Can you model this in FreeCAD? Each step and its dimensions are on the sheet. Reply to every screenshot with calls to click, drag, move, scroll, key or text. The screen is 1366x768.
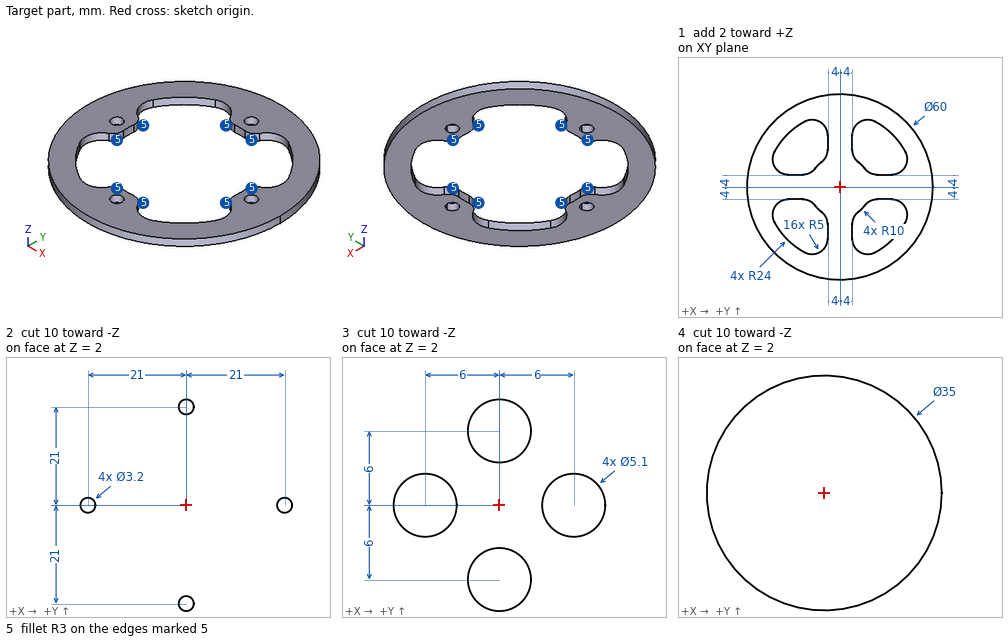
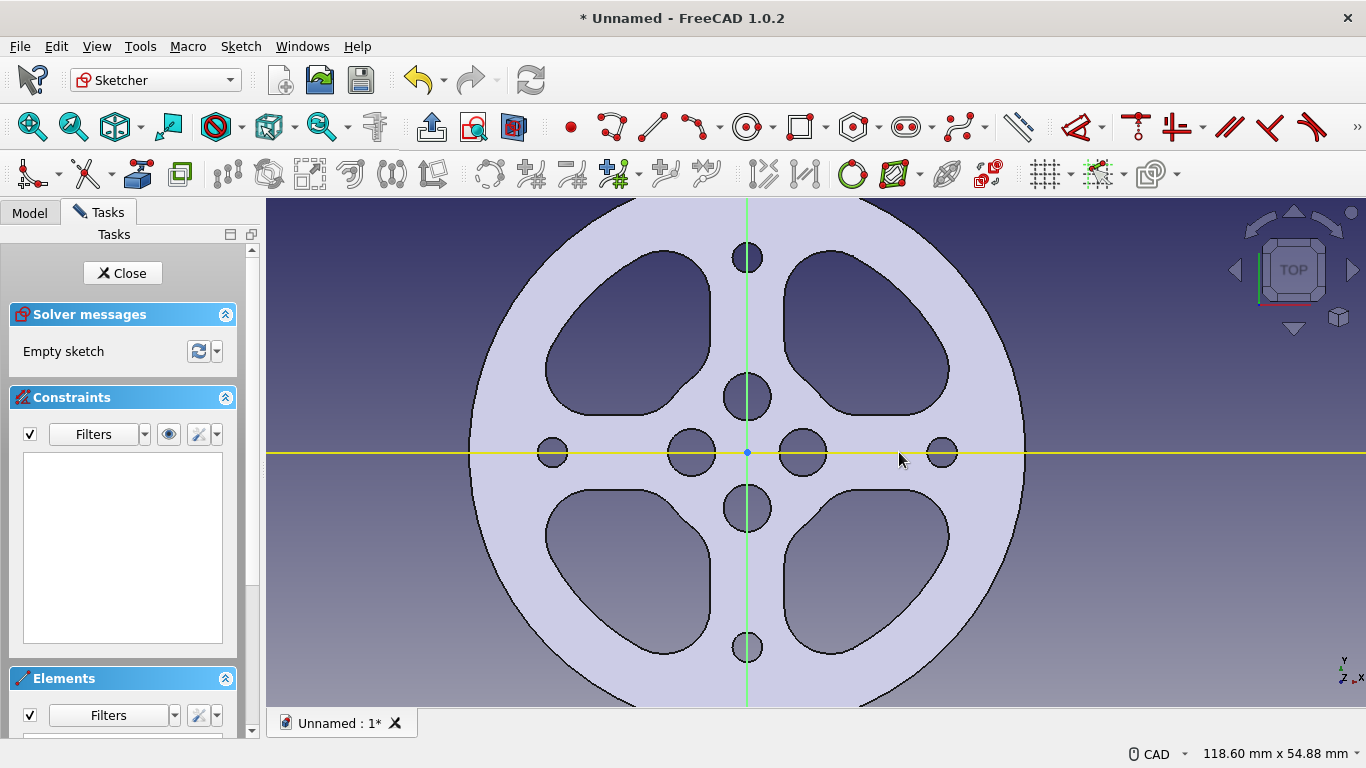
click(746, 128)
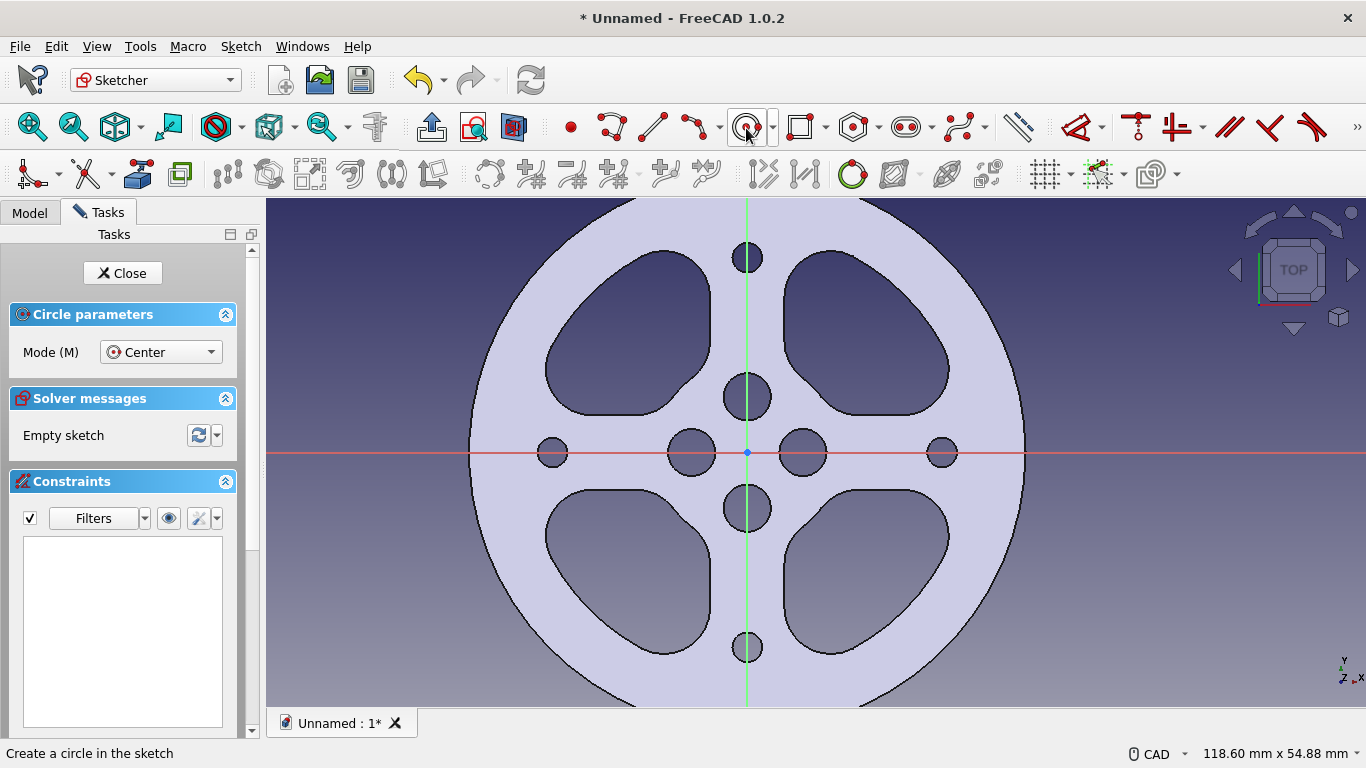
click(747, 452)
click(862, 338)
key(Escape)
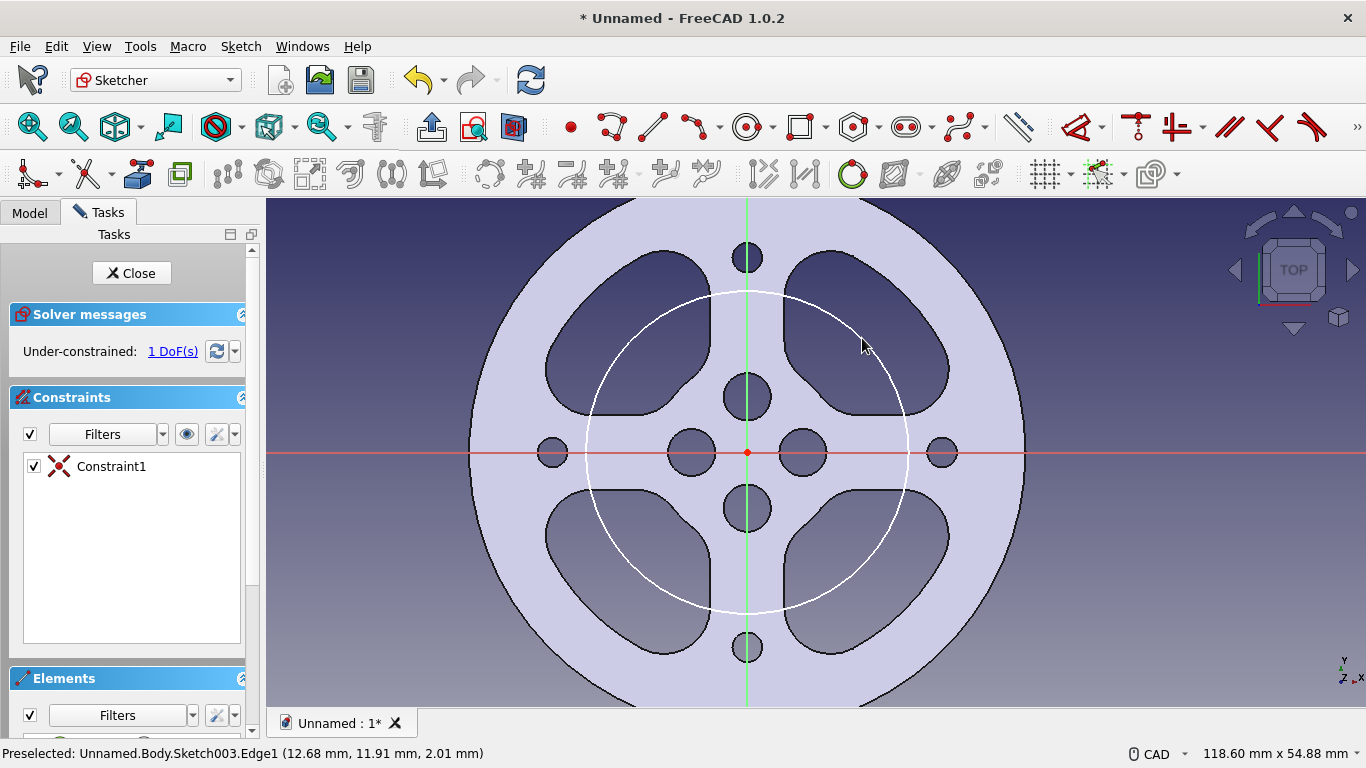
key(d)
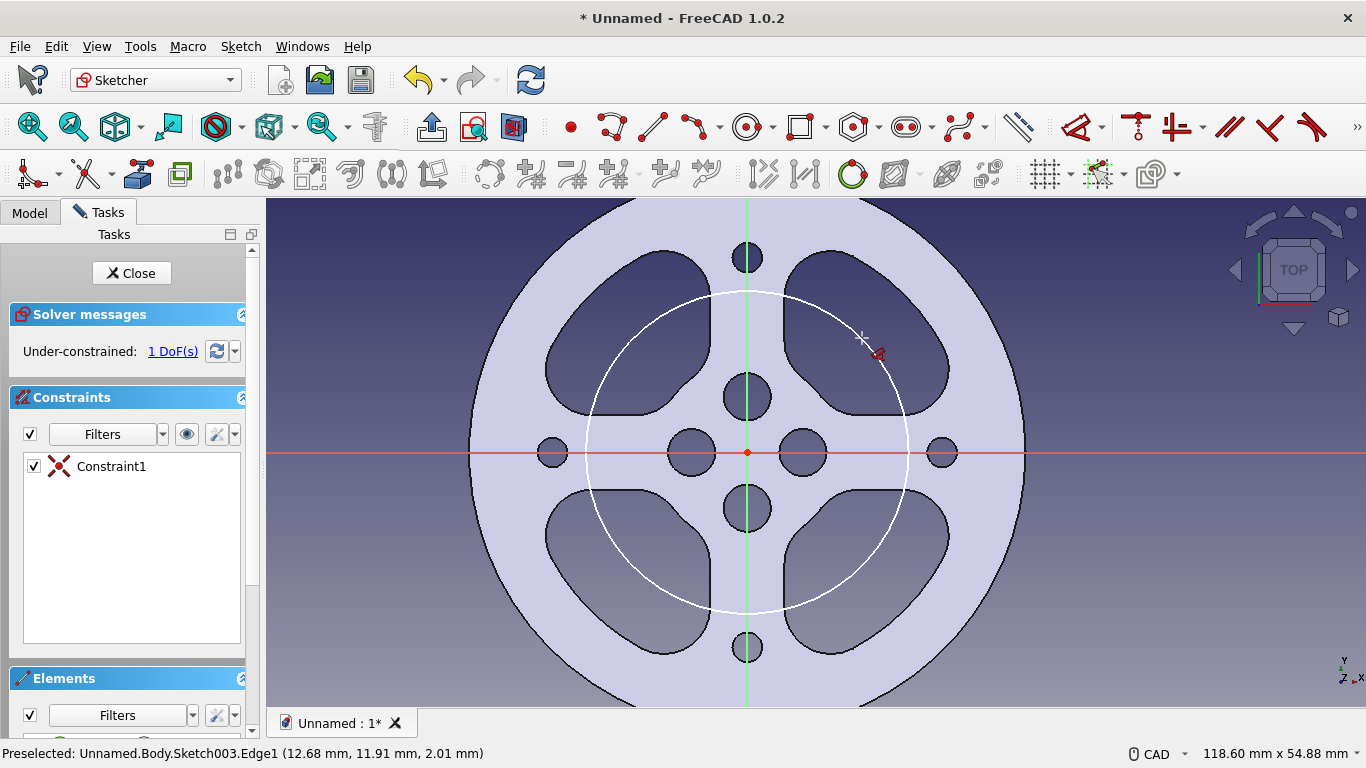
click(861, 338)
click(884, 315)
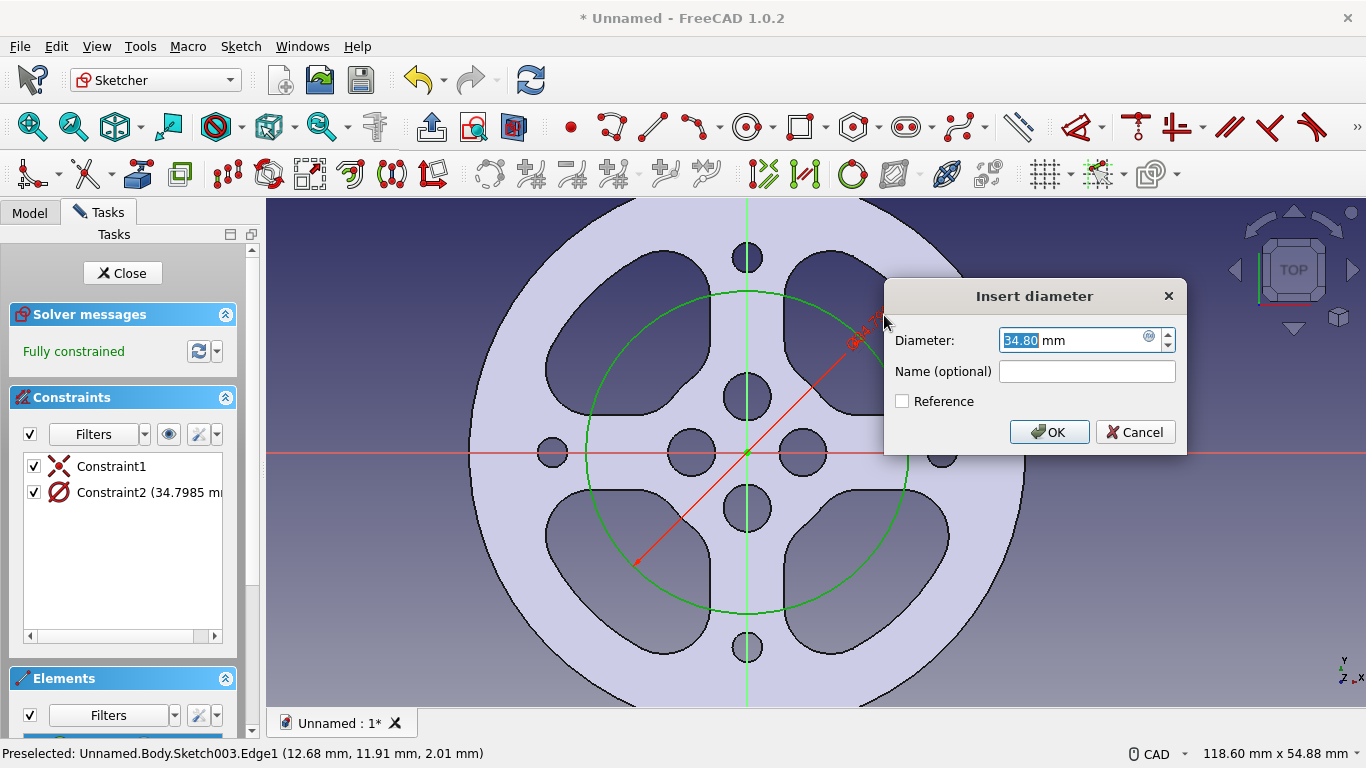
text(35)
key(Return)
key(Escape)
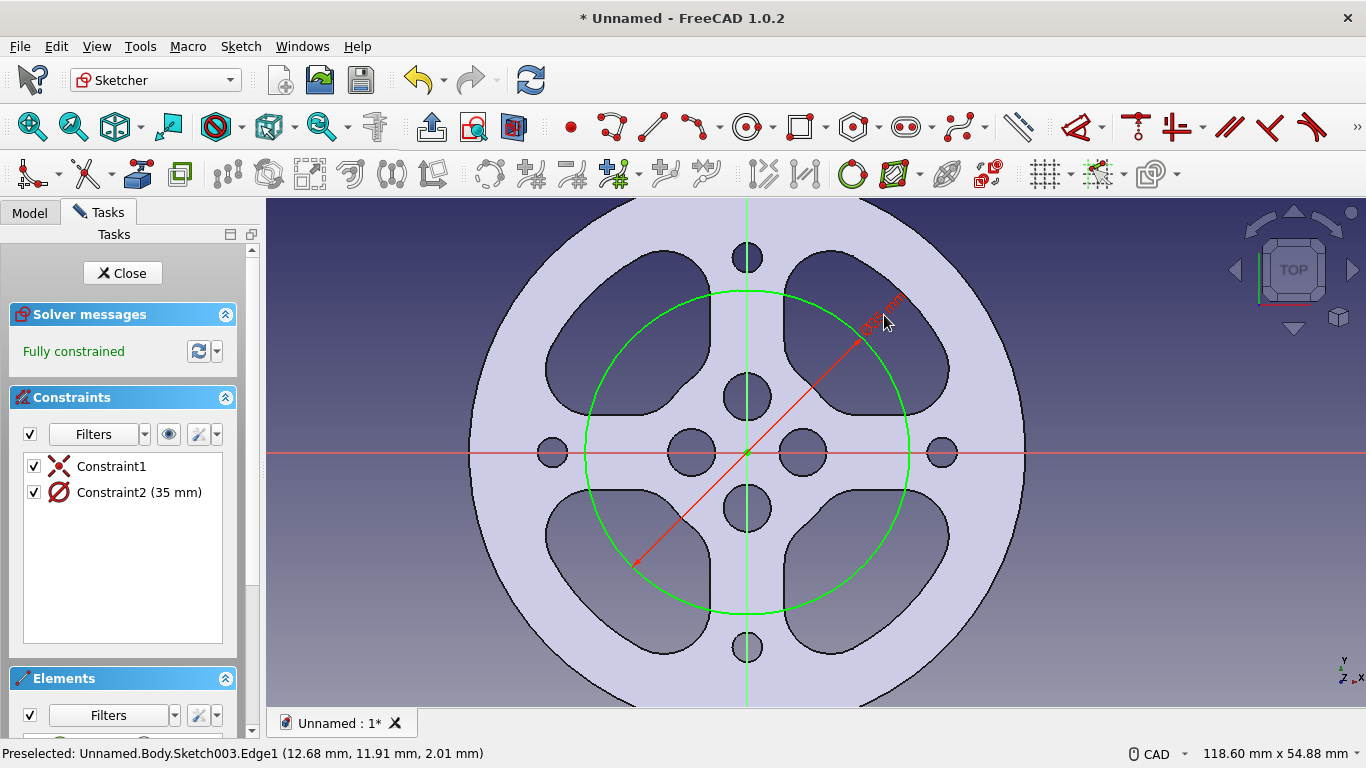
click(123, 273)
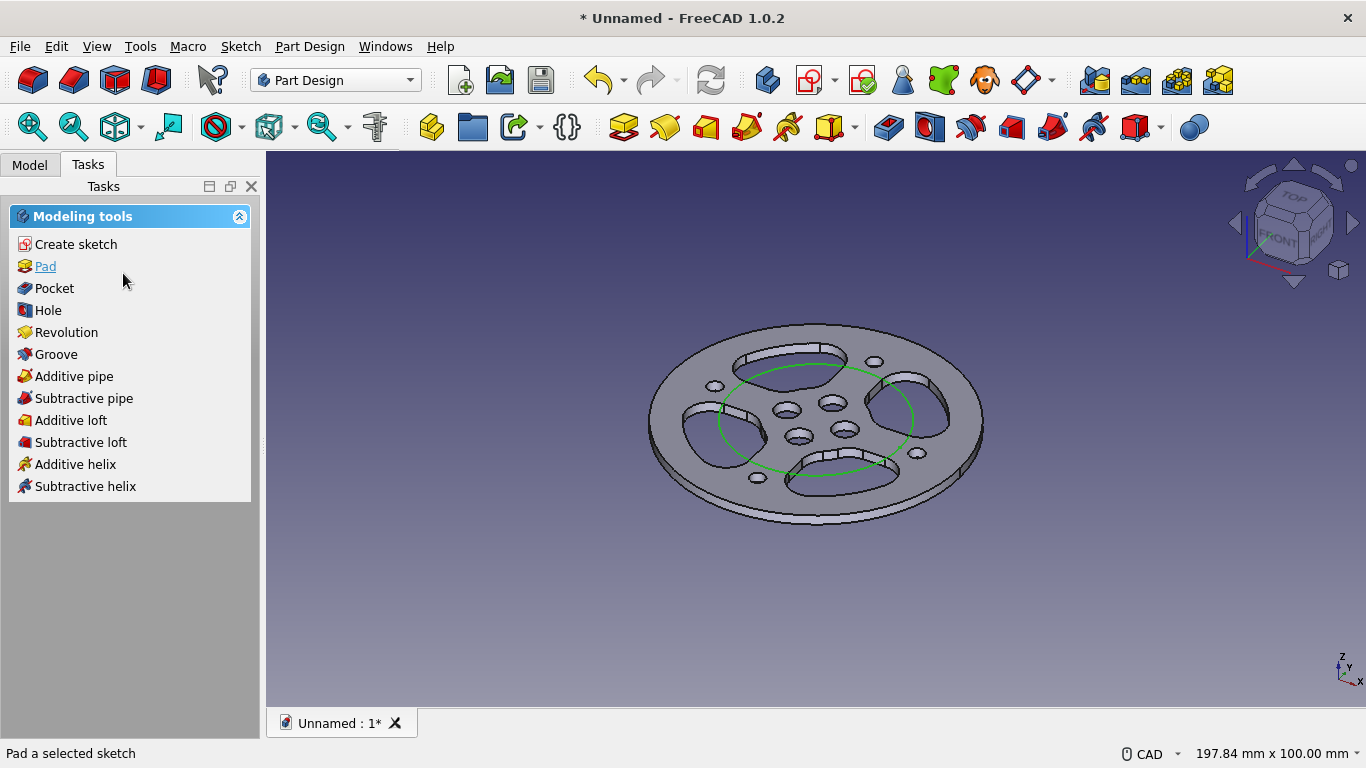
click(889, 128)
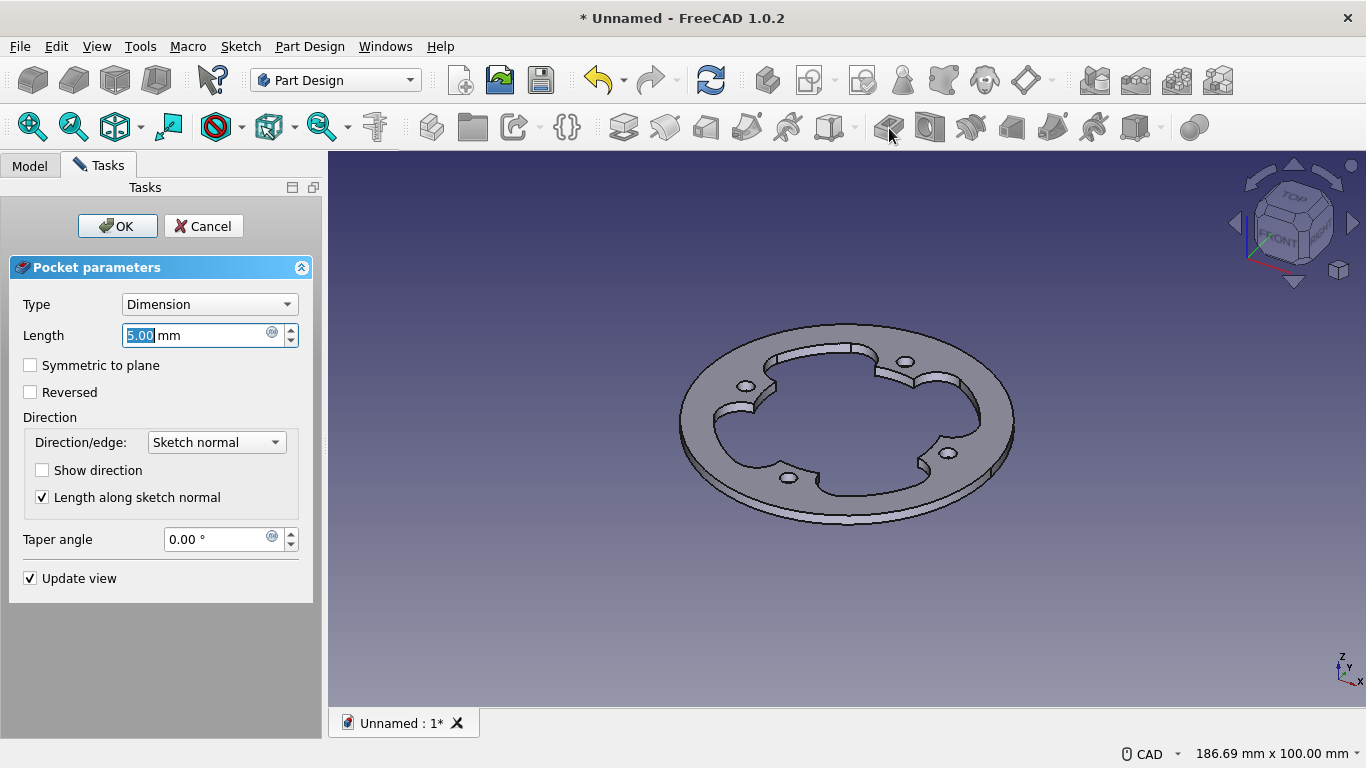
text(10)
key(Tab)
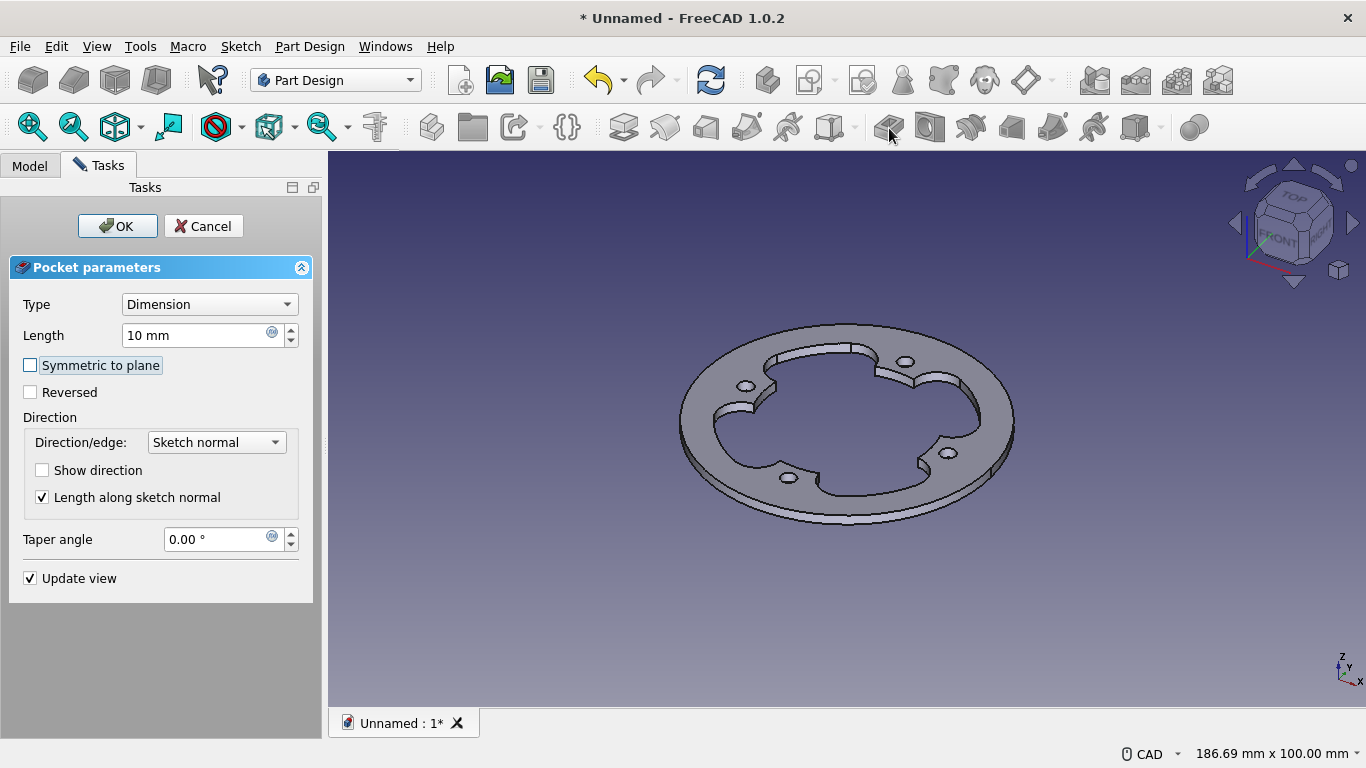
click(118, 226)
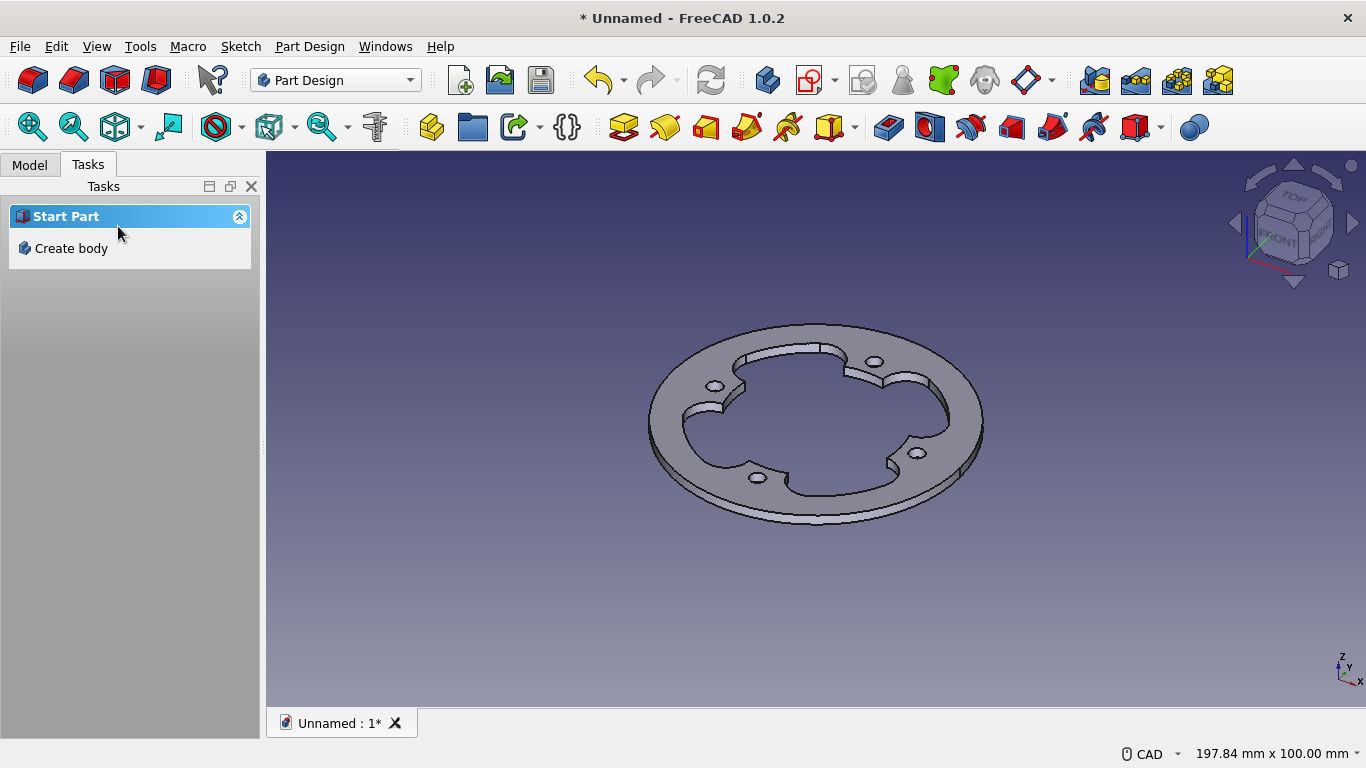
click(883, 385)